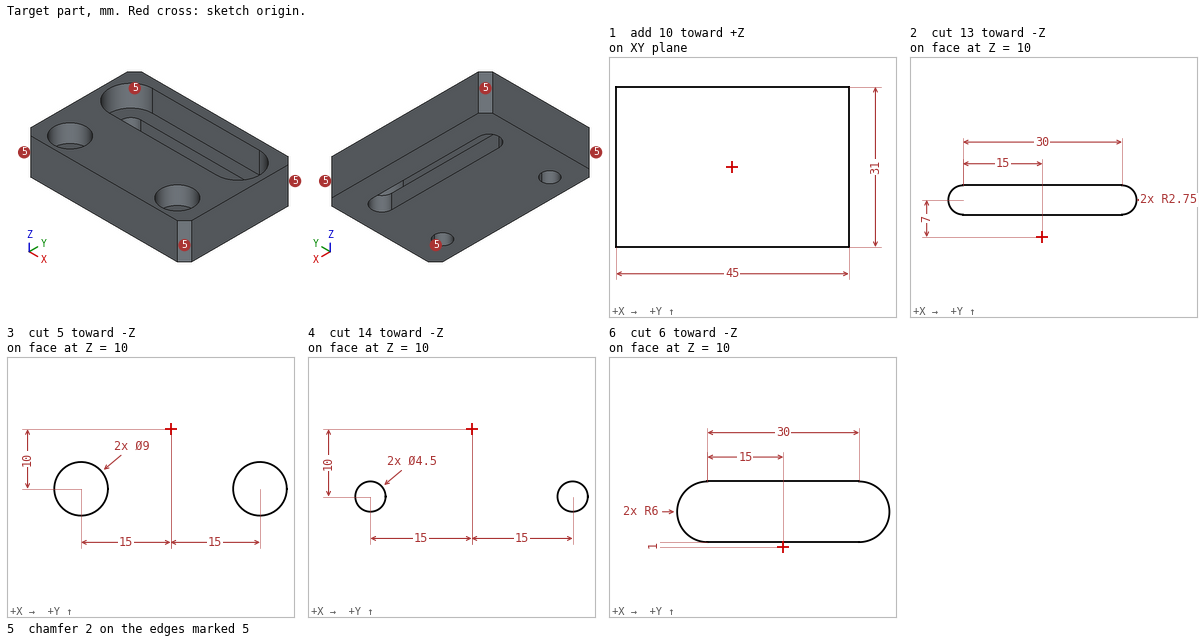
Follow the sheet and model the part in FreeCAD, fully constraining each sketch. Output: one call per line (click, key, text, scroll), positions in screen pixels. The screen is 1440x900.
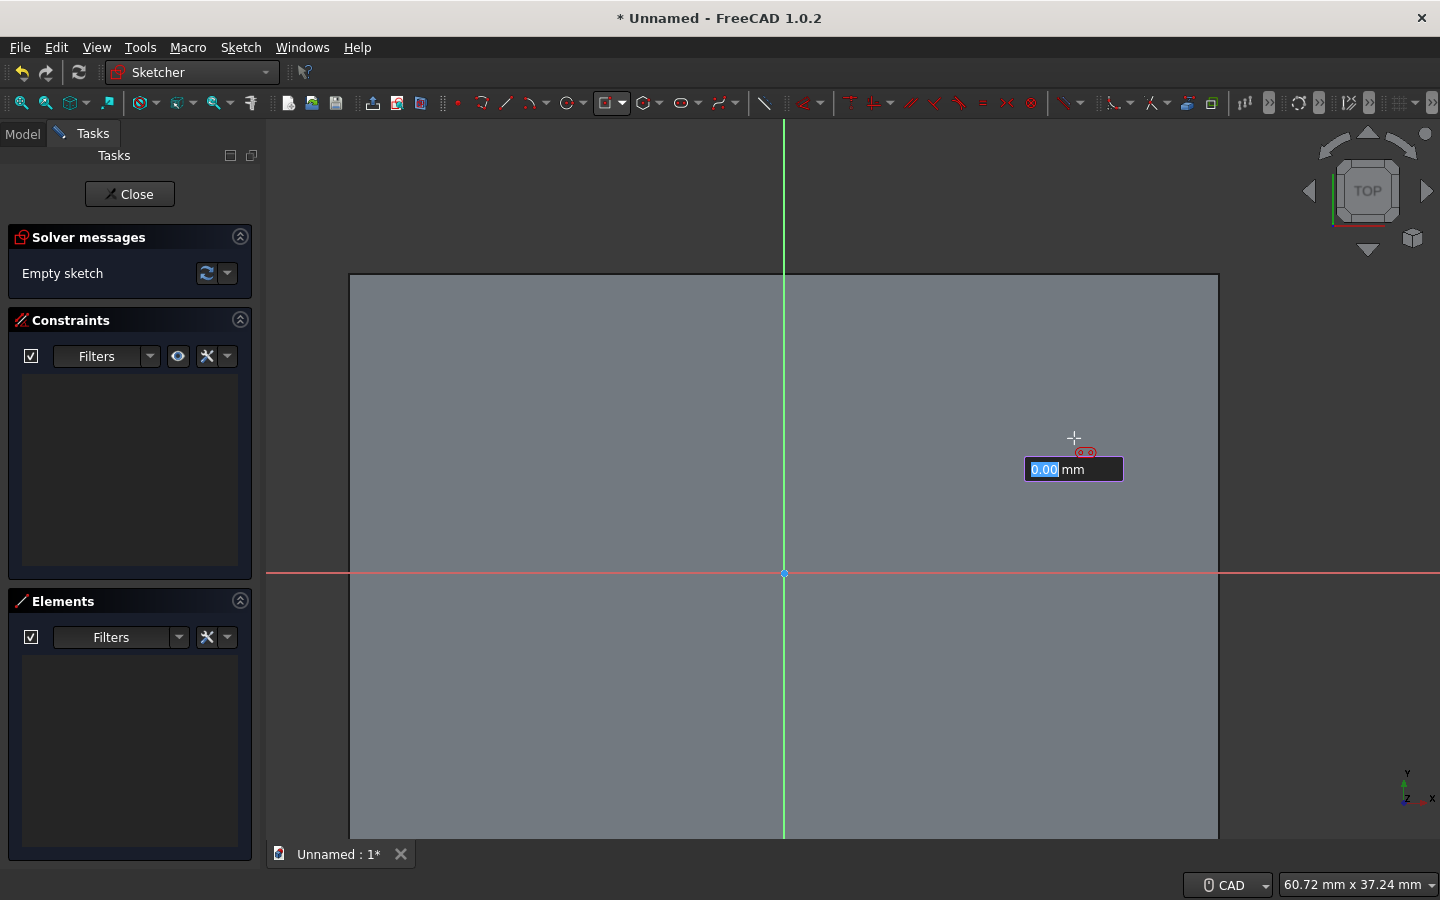
click(871, 385)
key(Escape)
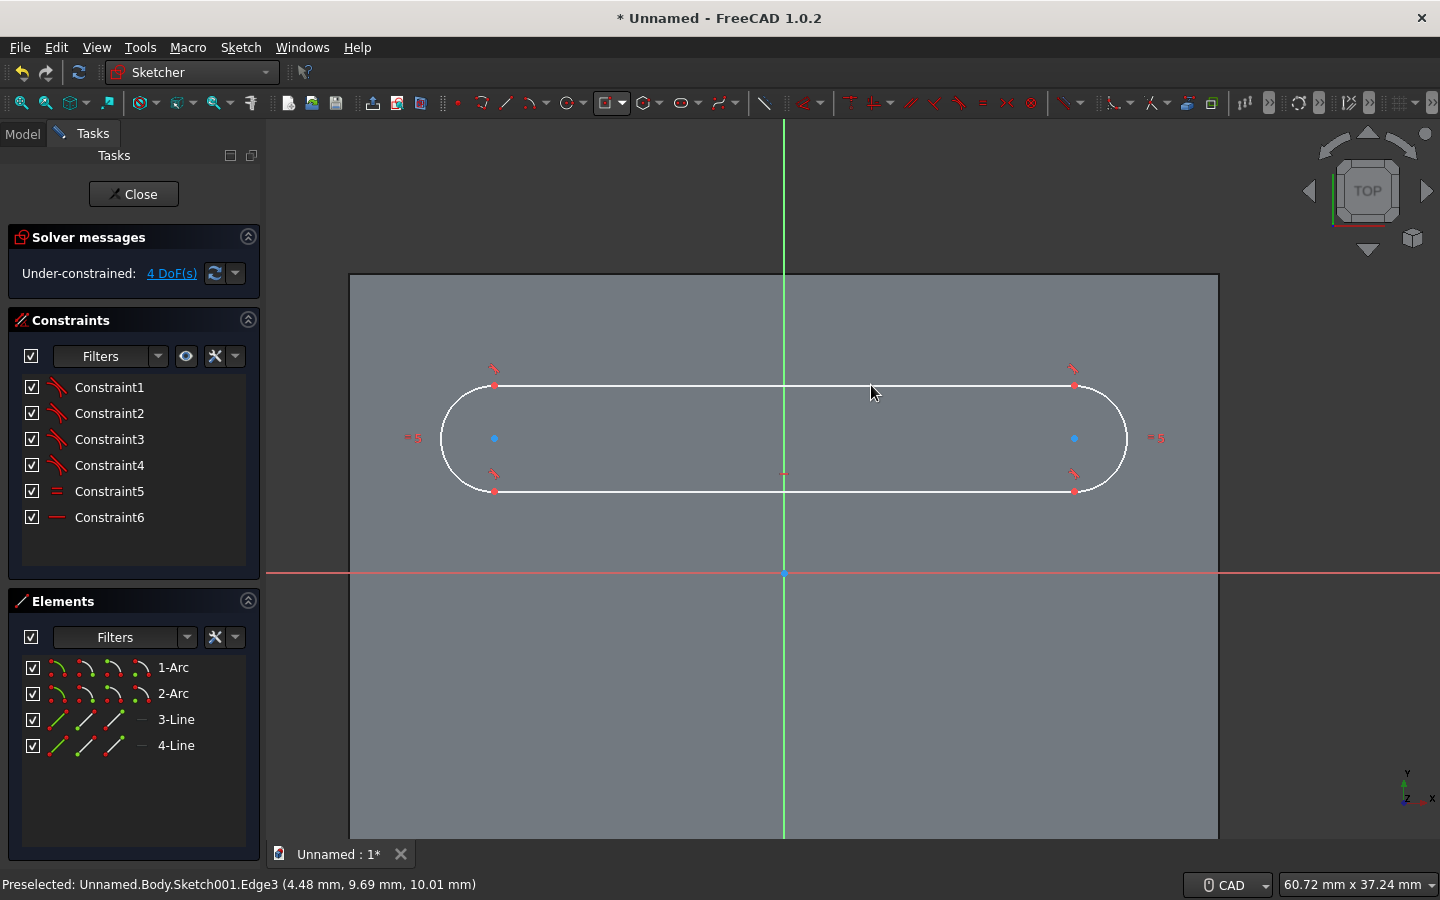
click(804, 104)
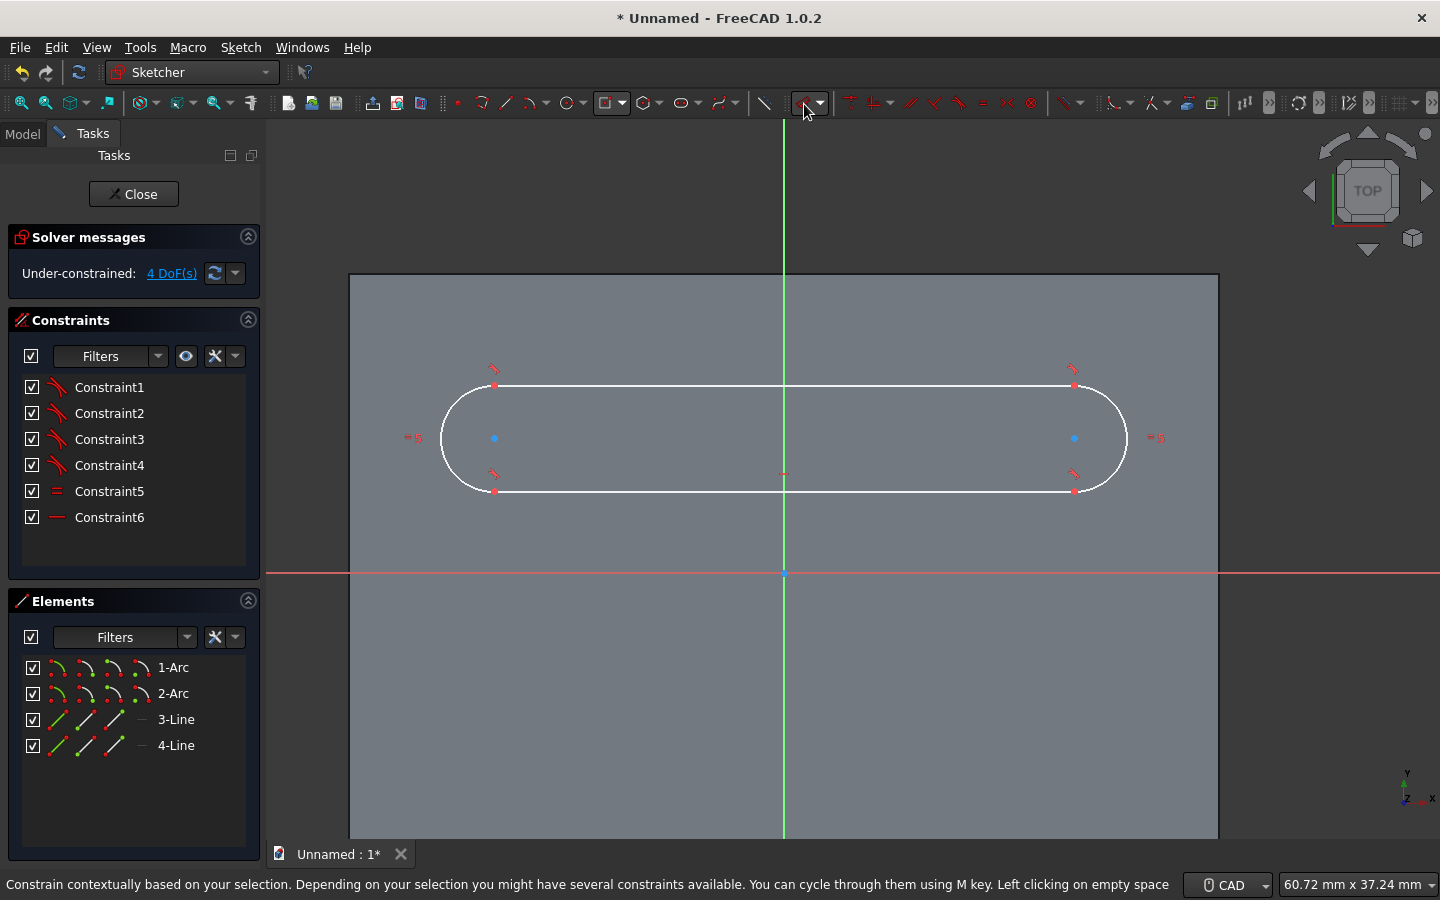
click(451, 408)
click(425, 389)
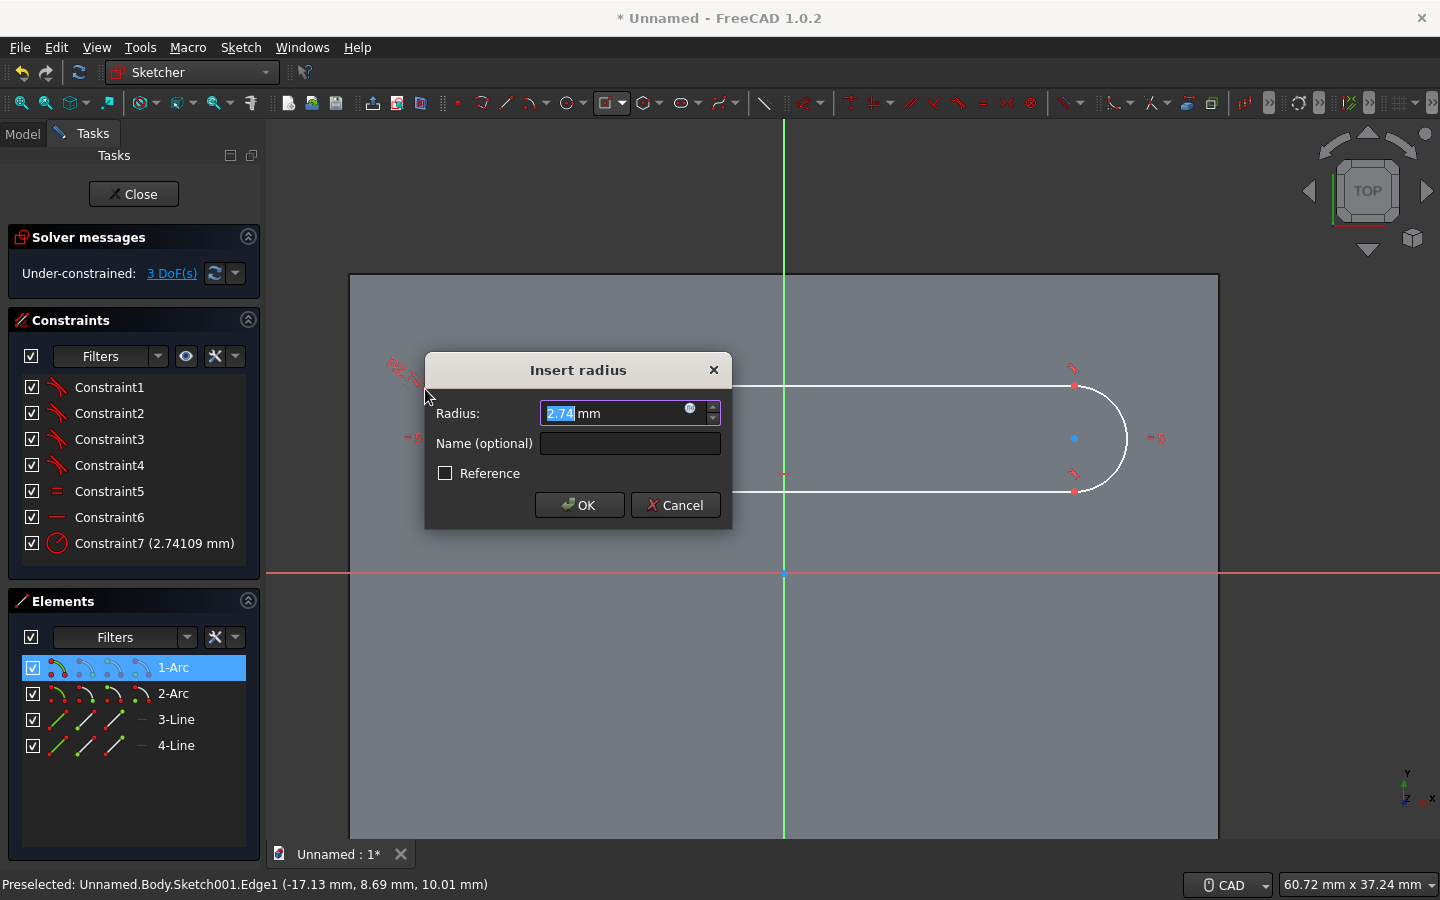
text(2.75)
key(Return)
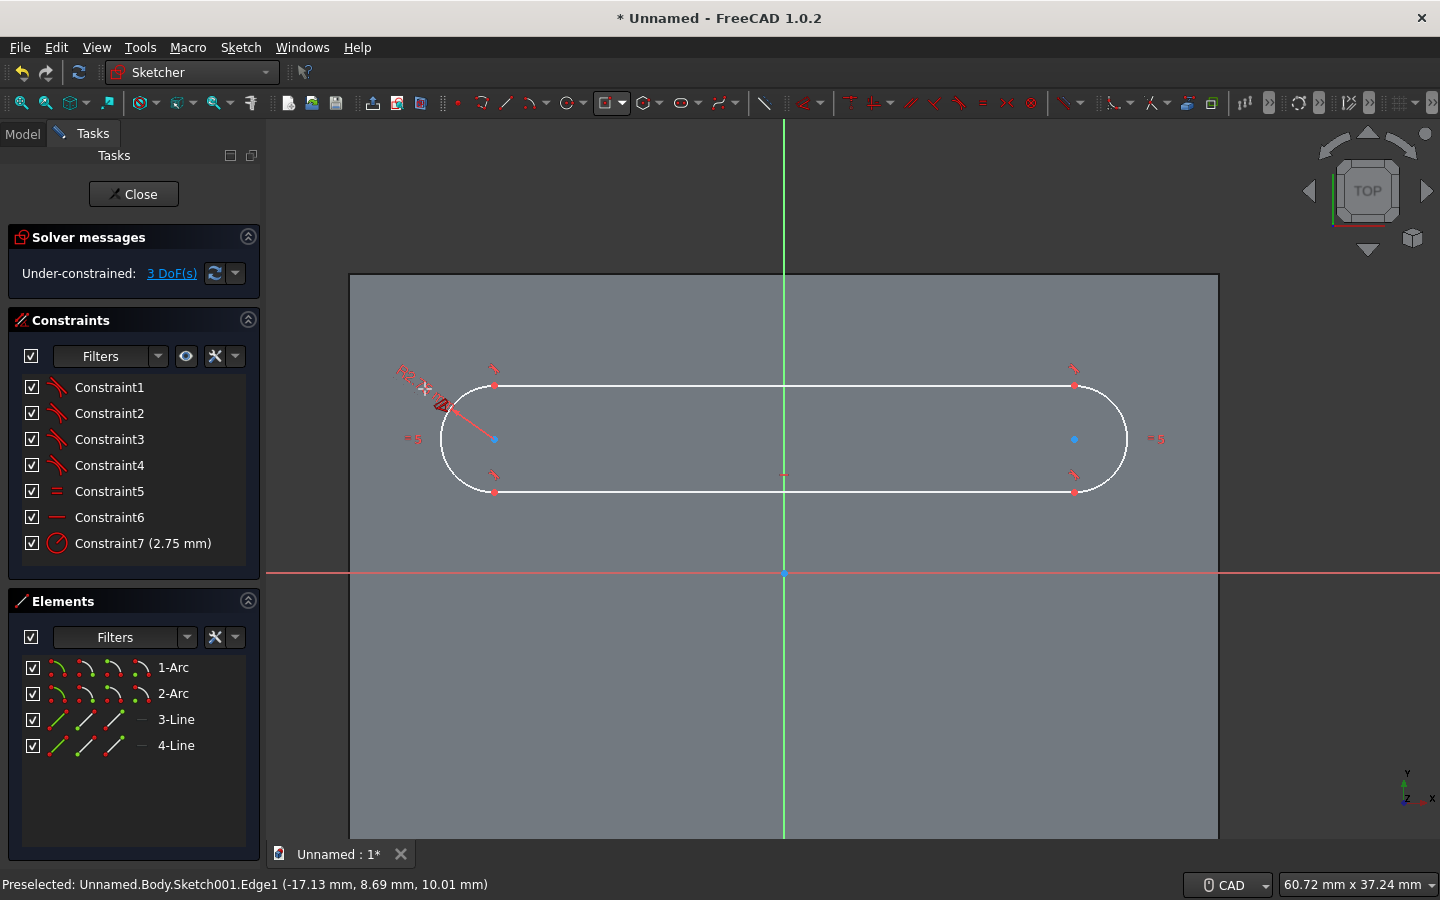
click(668, 386)
click(651, 352)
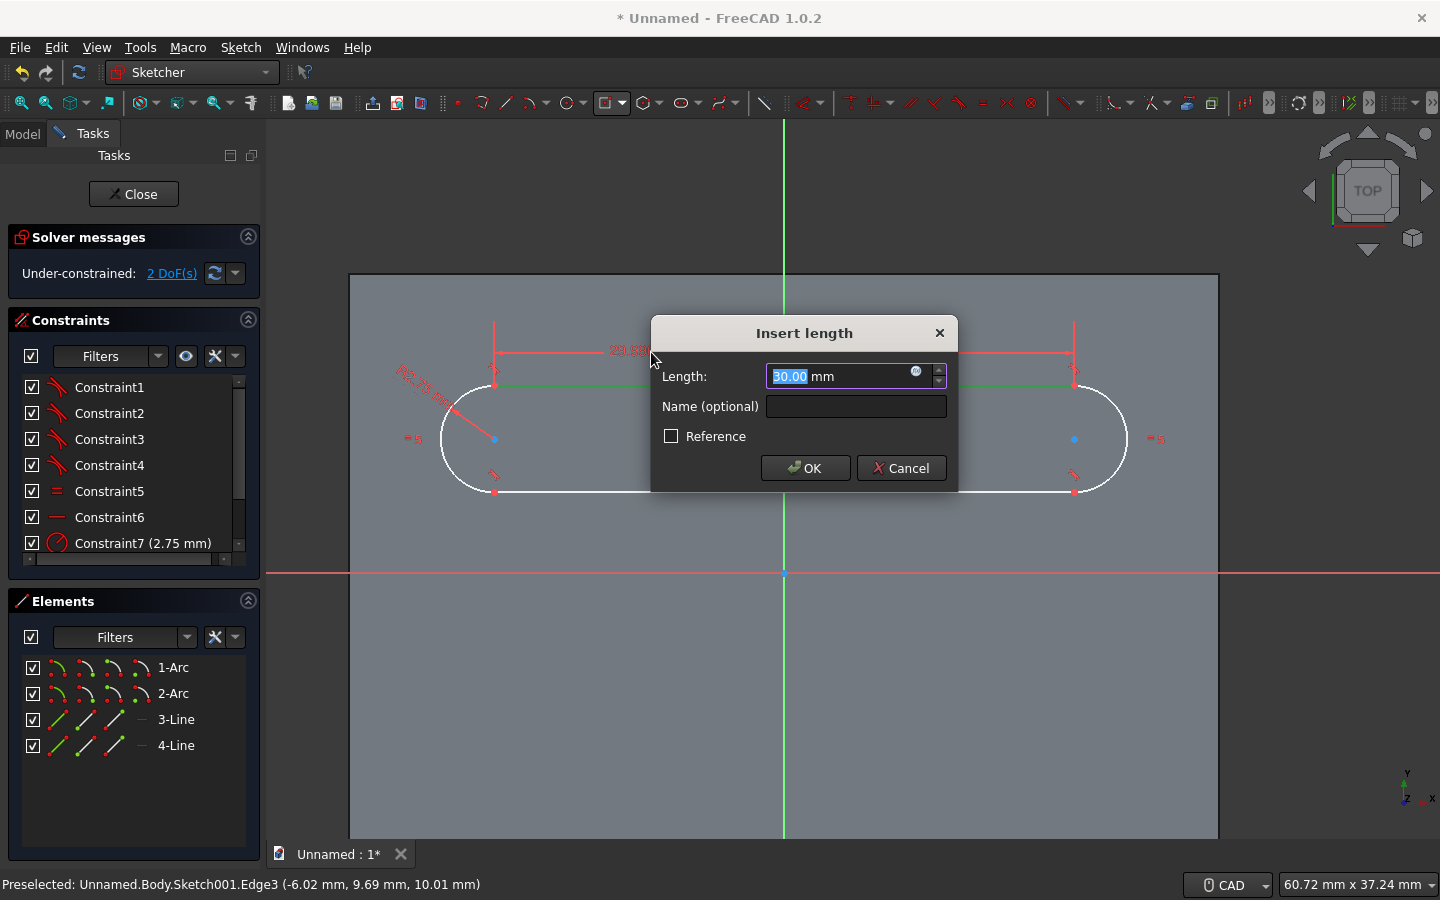
text(30)
key(Return)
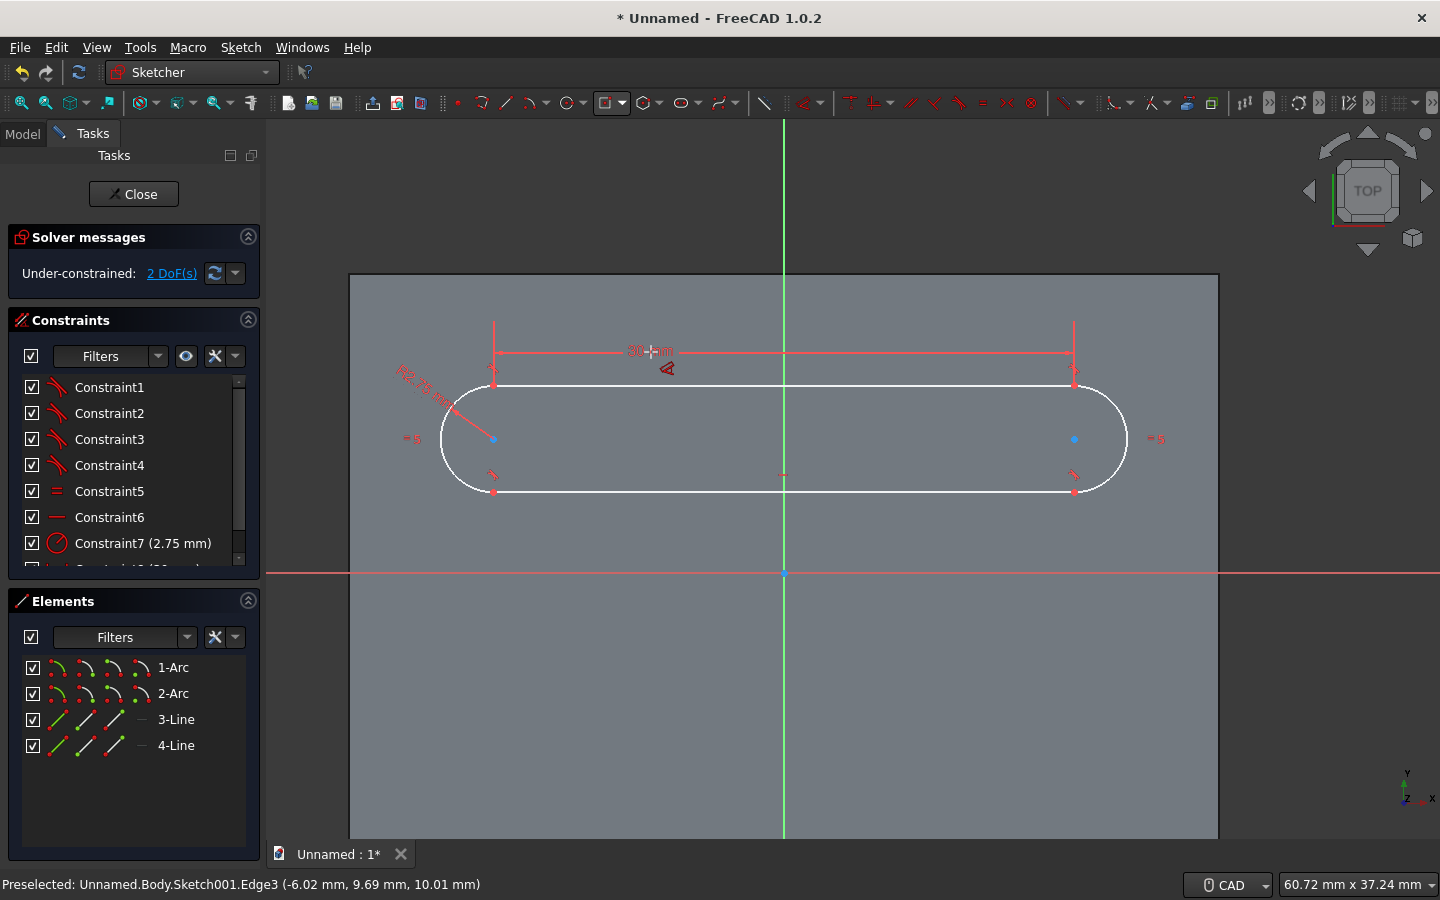
click(494, 439)
click(460, 506)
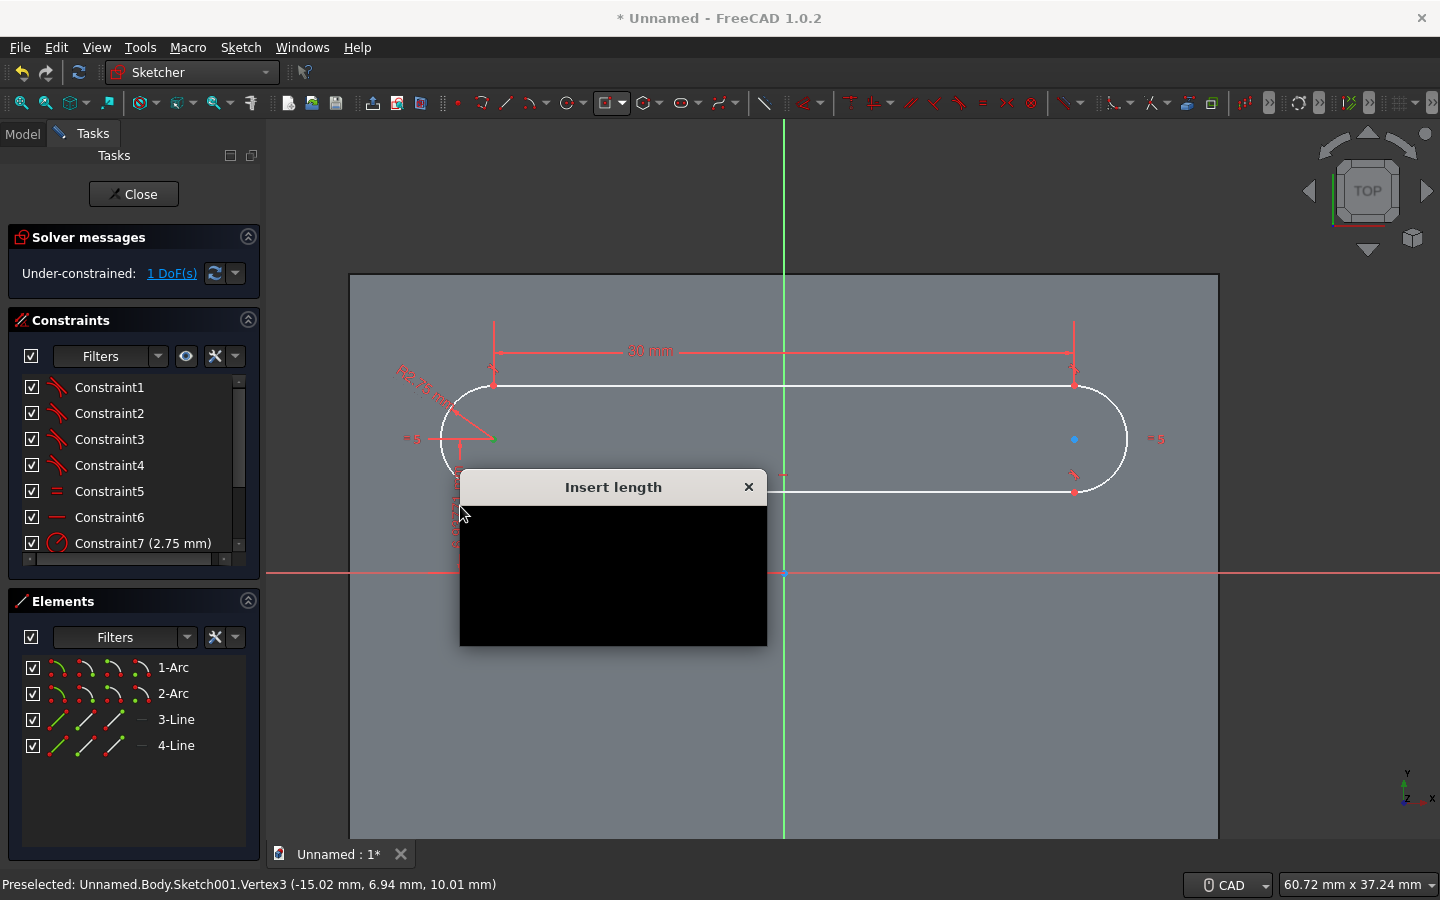
text(7)
key(Return)